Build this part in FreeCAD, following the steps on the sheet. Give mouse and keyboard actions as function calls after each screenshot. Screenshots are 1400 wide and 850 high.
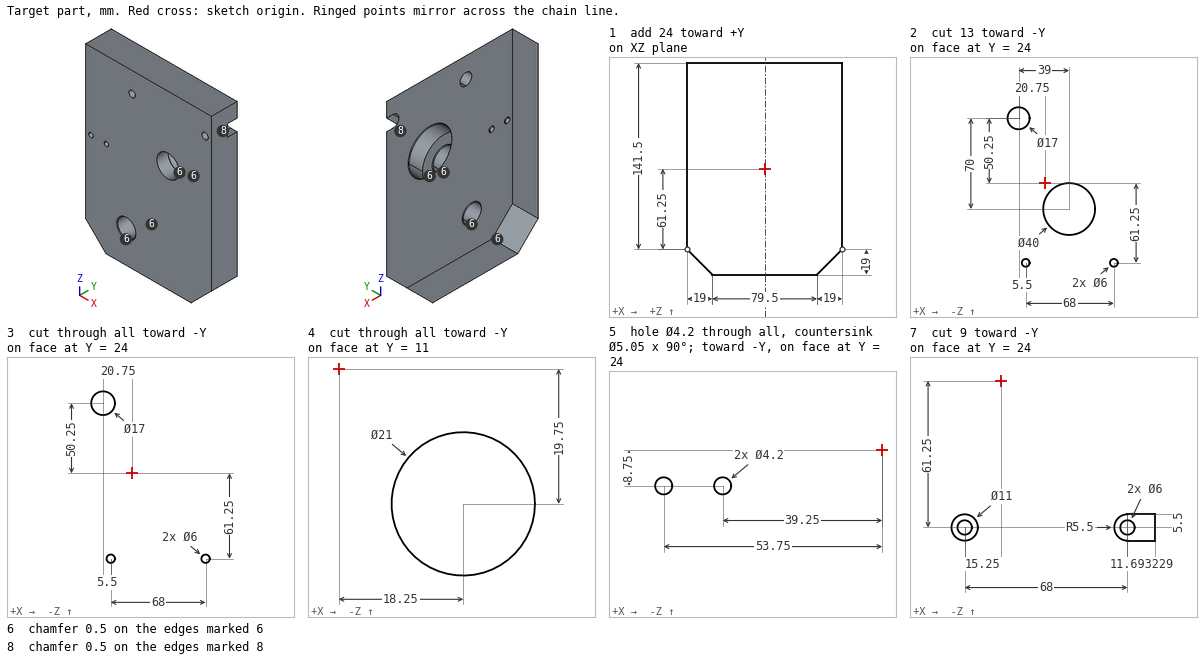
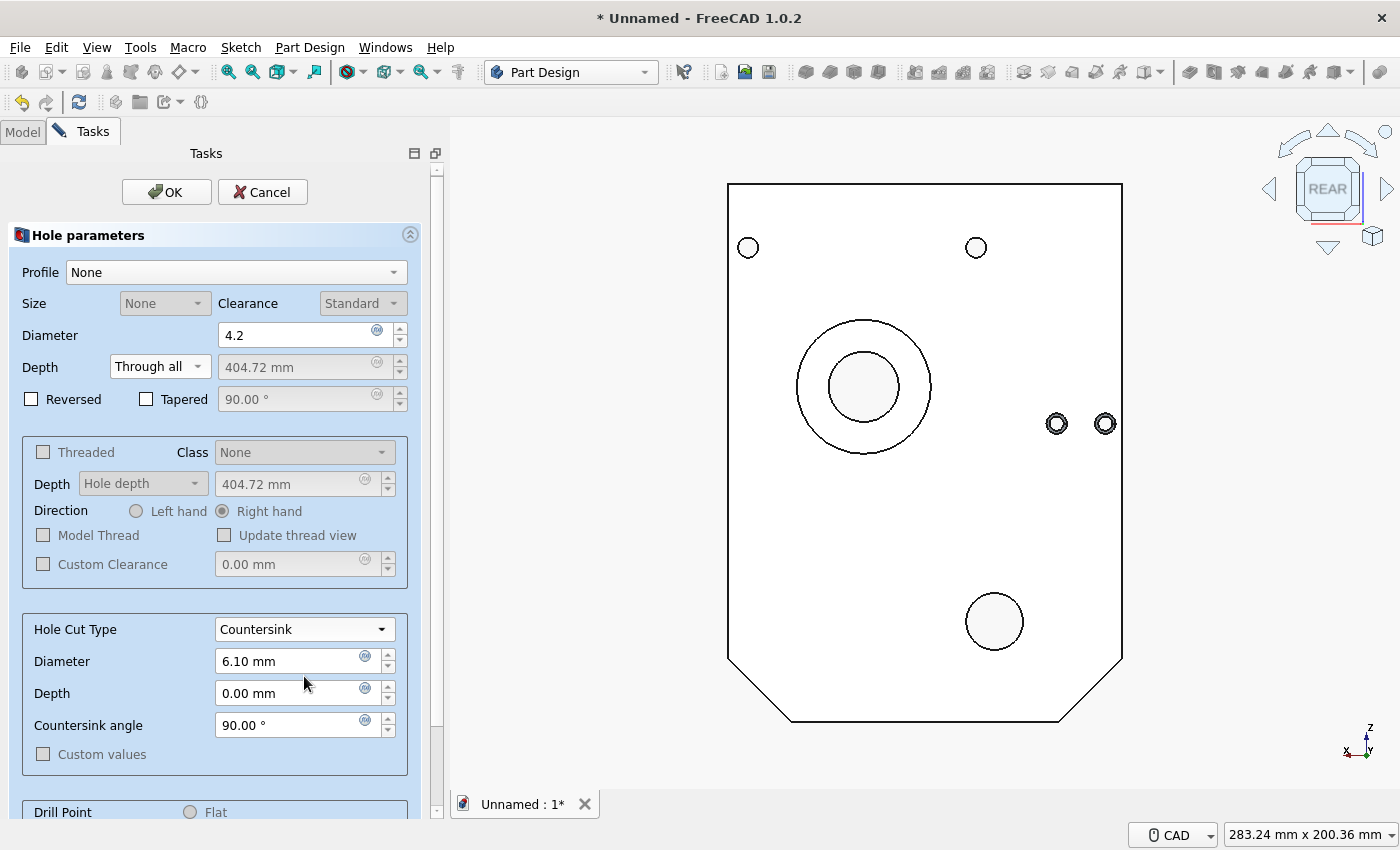
triple_click(298, 661)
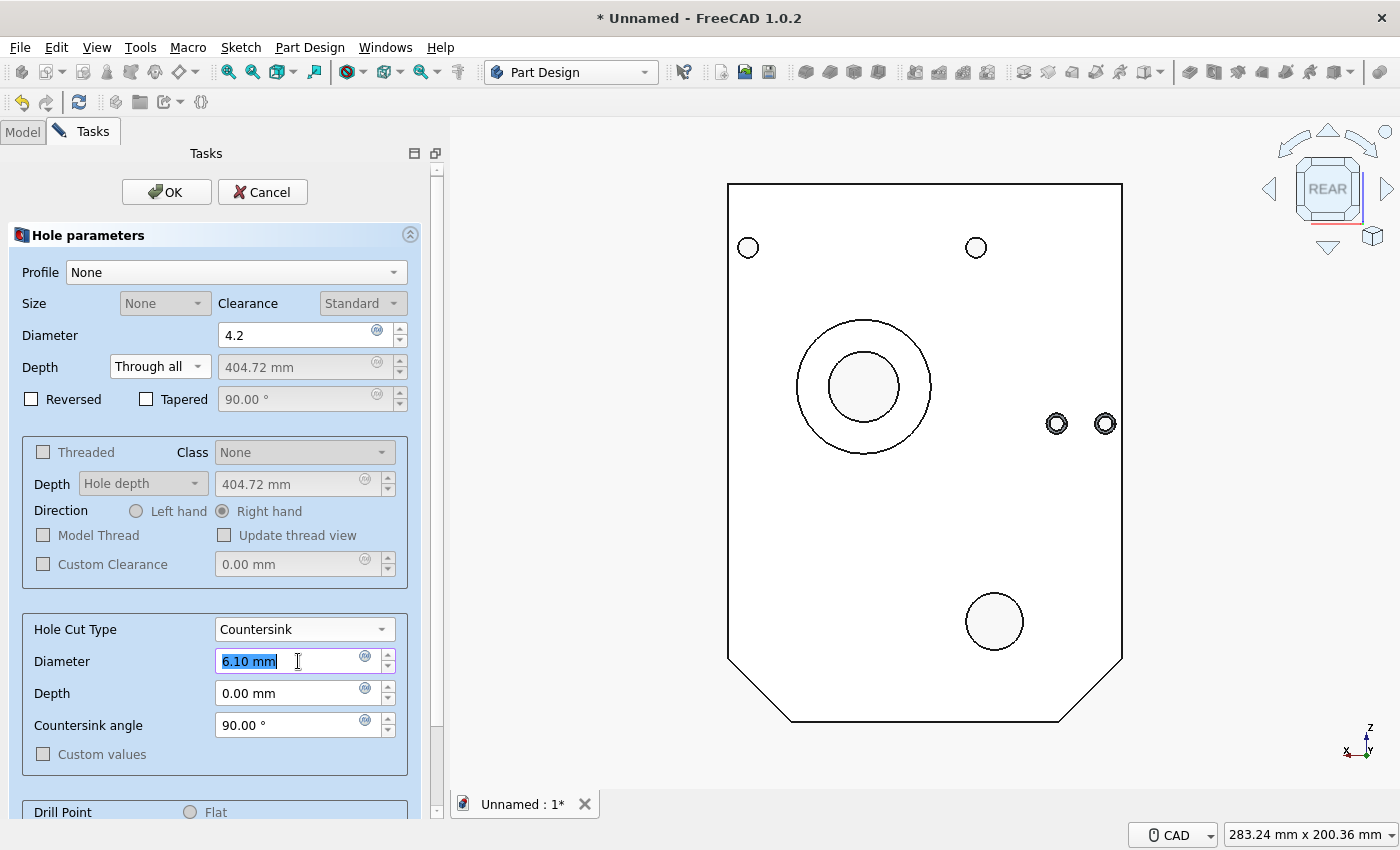
text(5.05)
key(Tab)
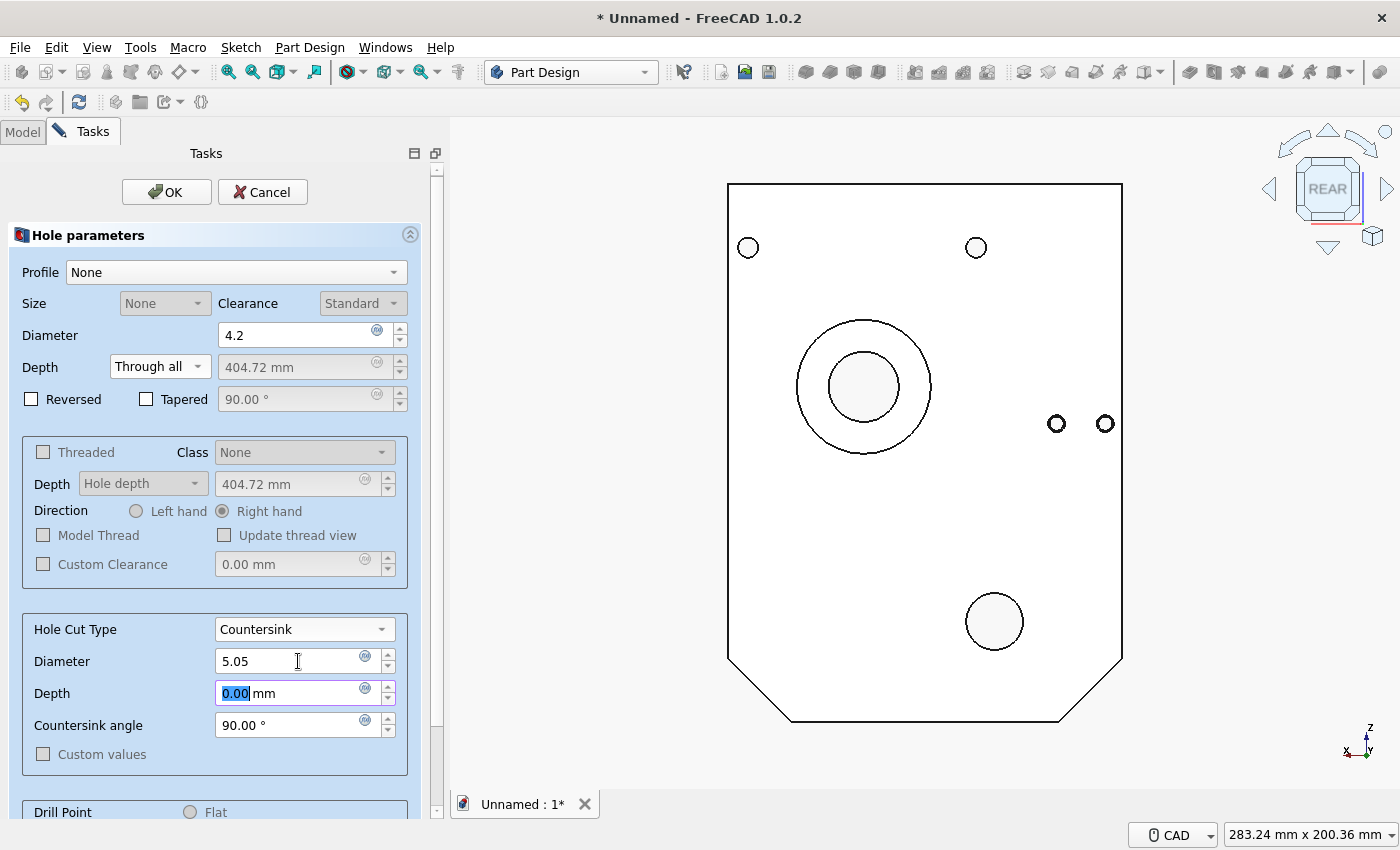
click(167, 192)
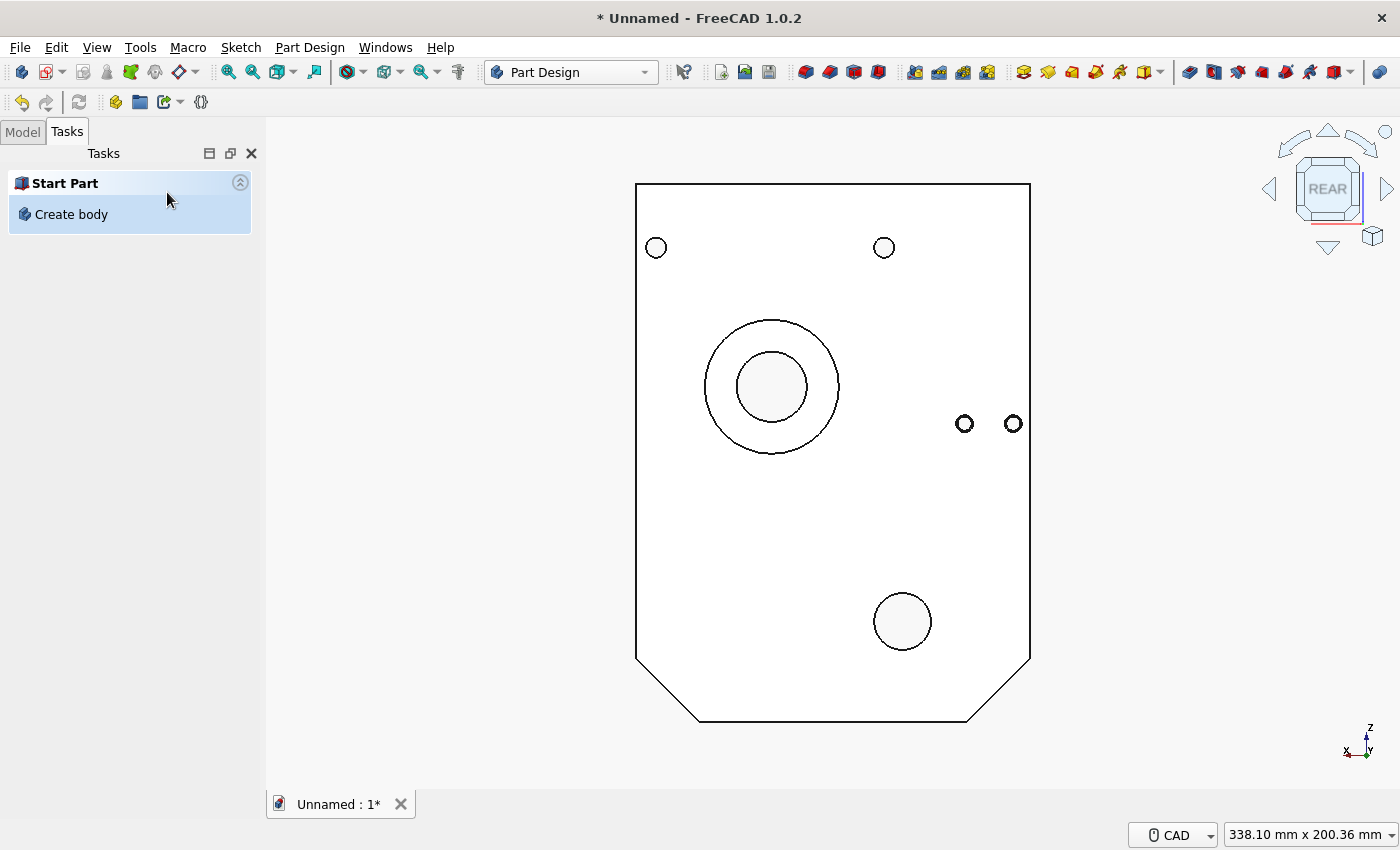
click(926, 604)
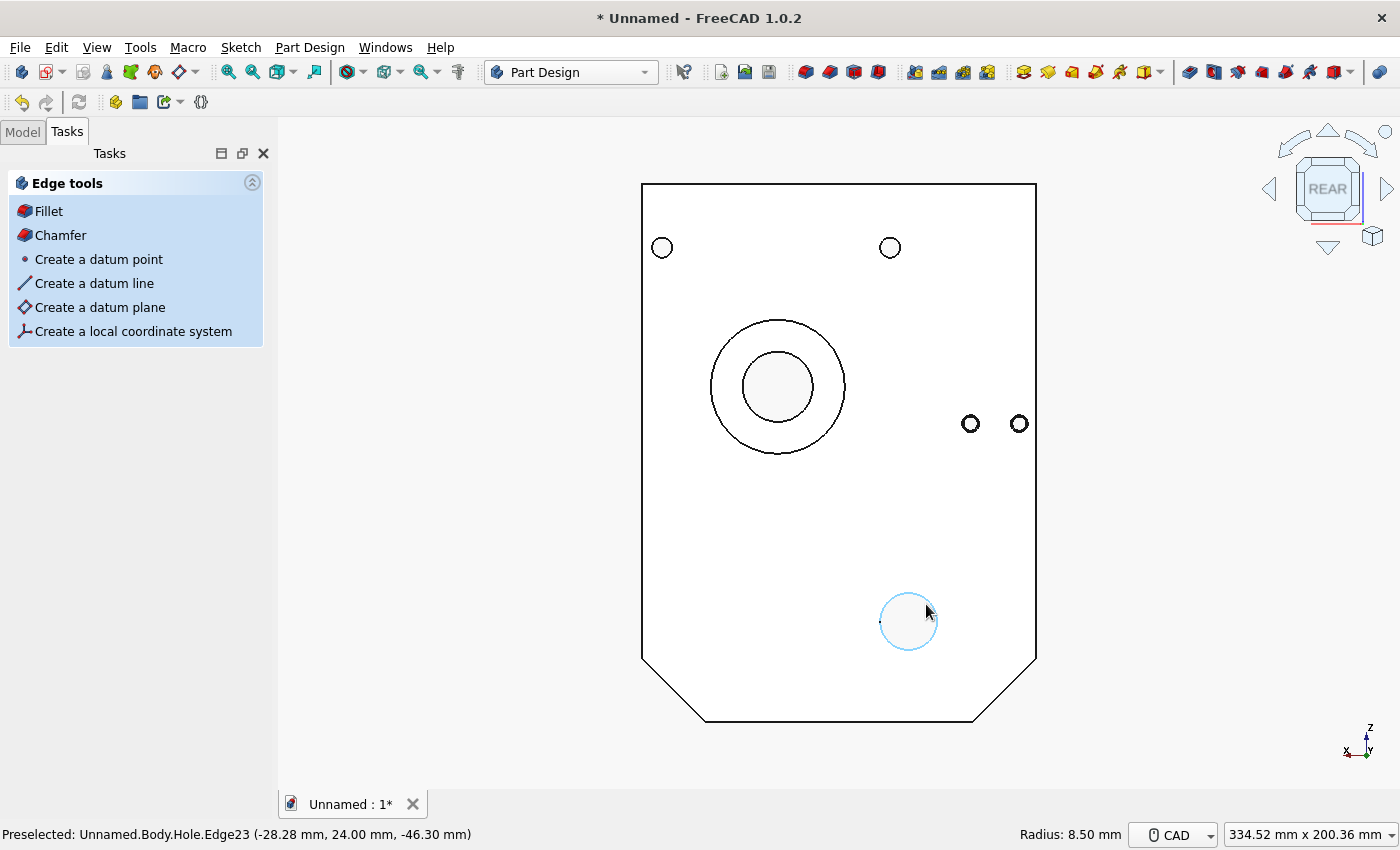
click(832, 346, ctrl)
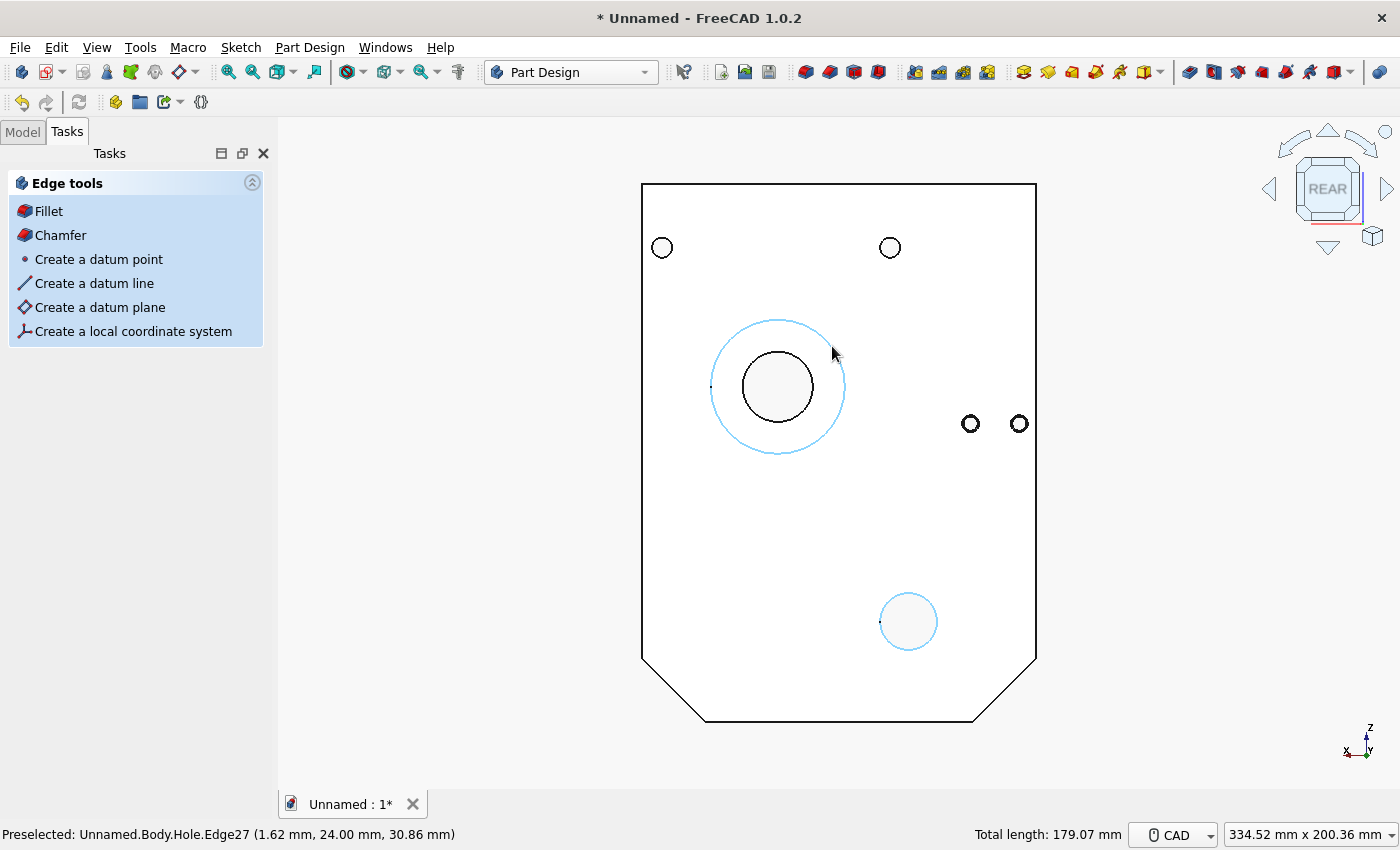
click(806, 365, ctrl)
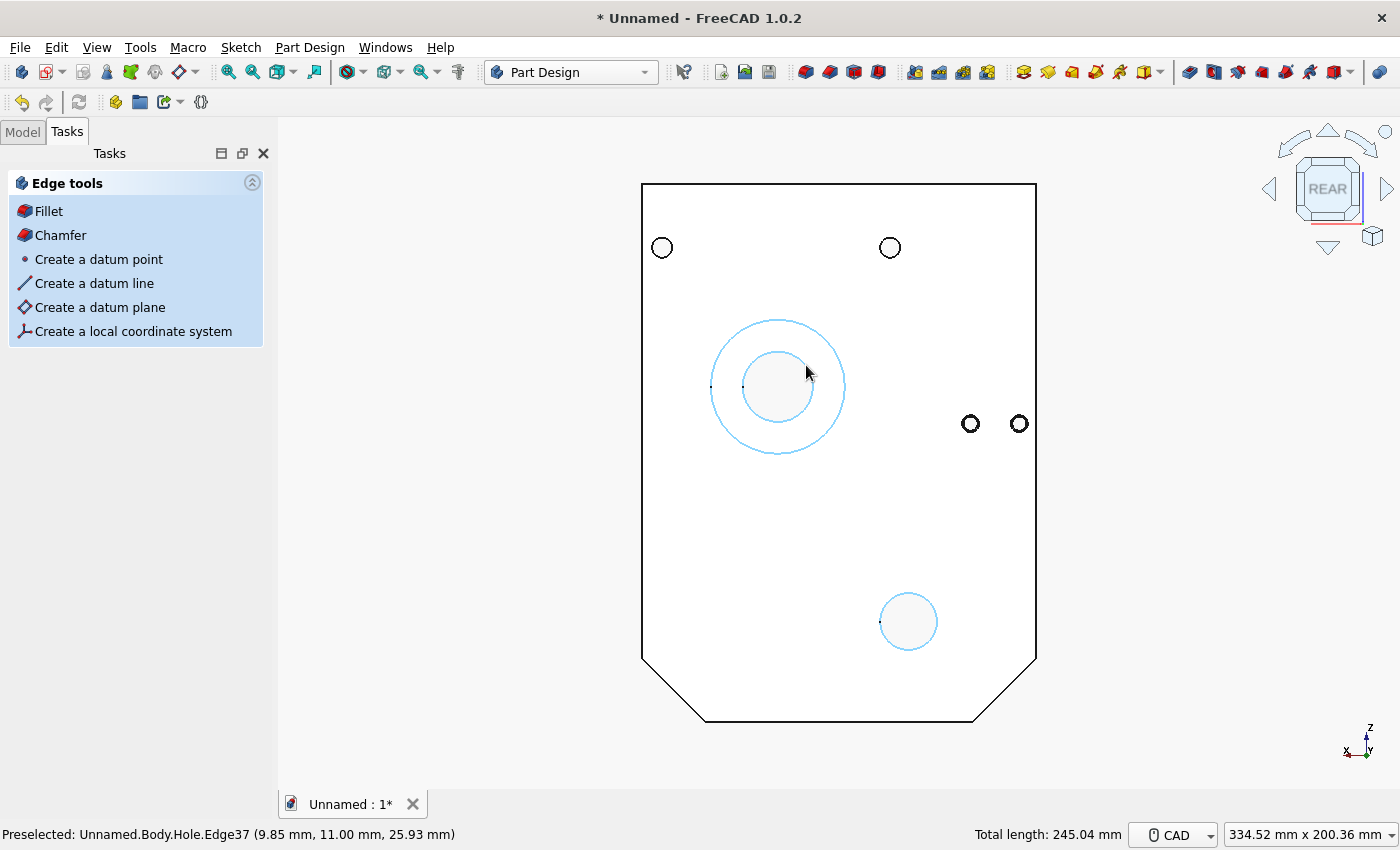
key(0)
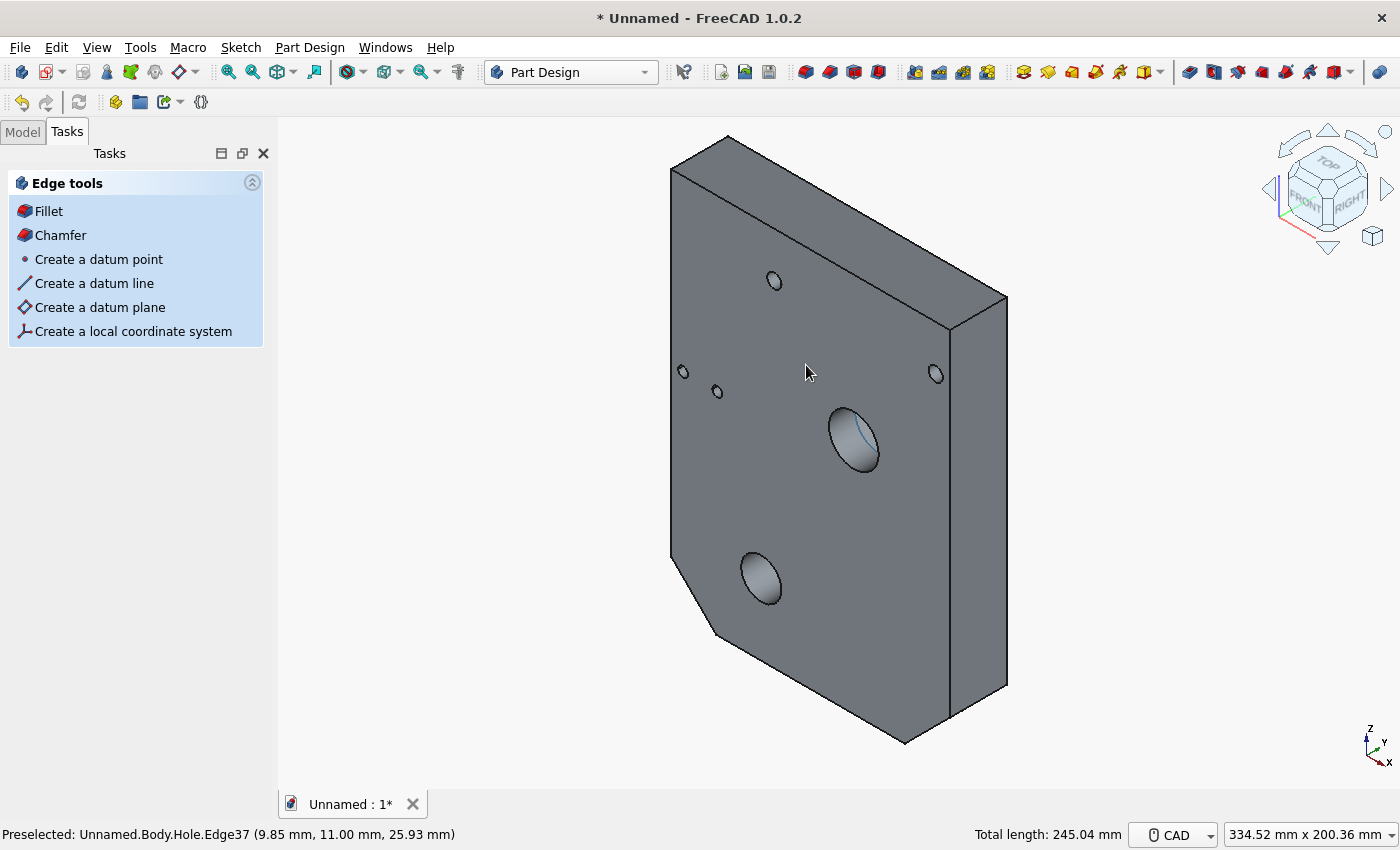
click(741, 566, ctrl)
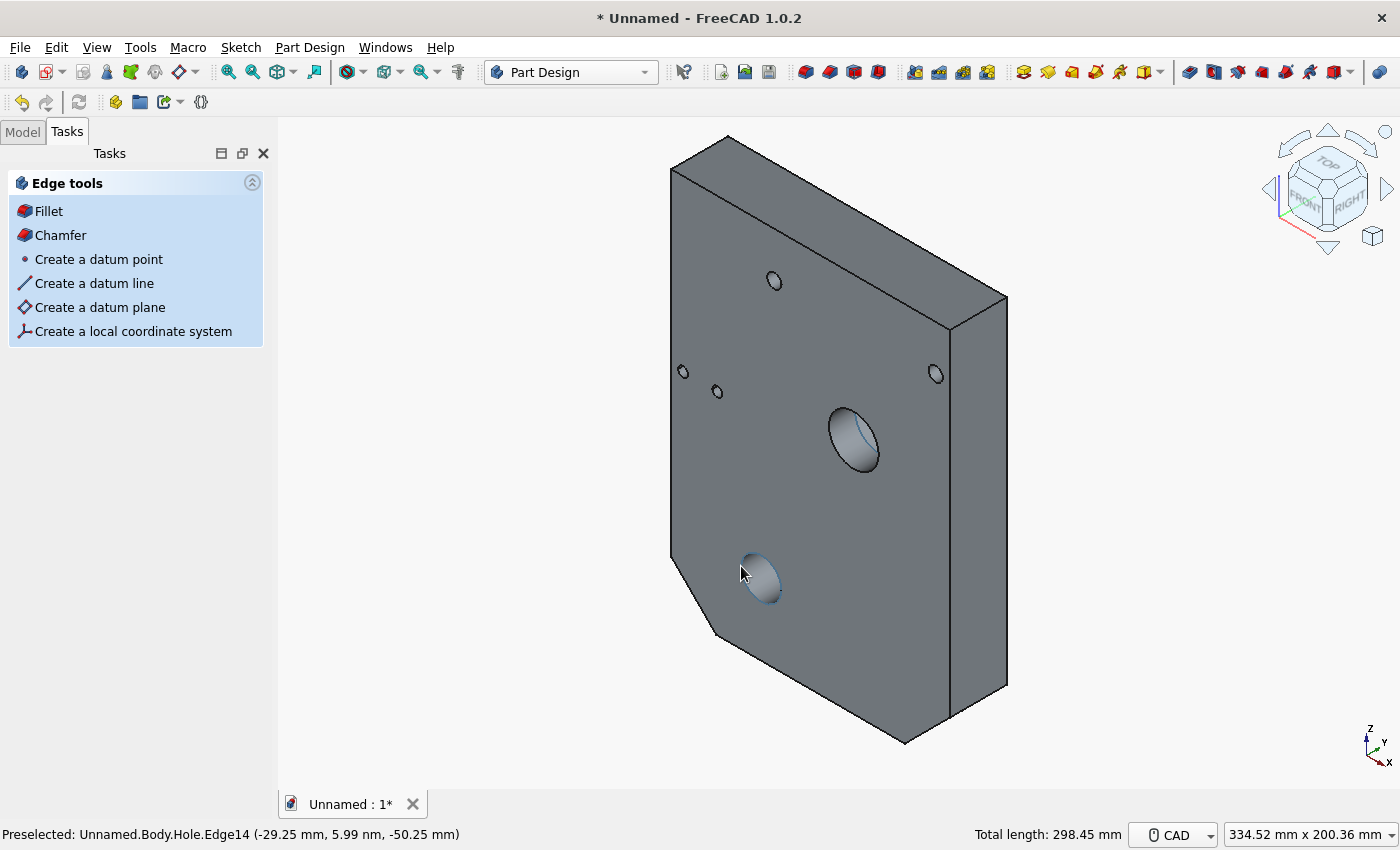
click(830, 72)